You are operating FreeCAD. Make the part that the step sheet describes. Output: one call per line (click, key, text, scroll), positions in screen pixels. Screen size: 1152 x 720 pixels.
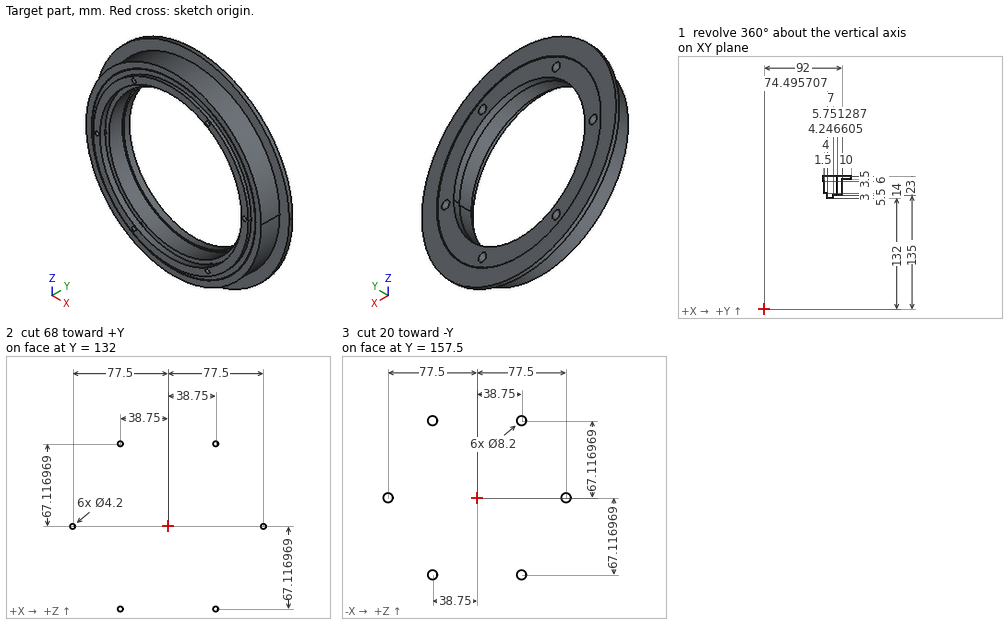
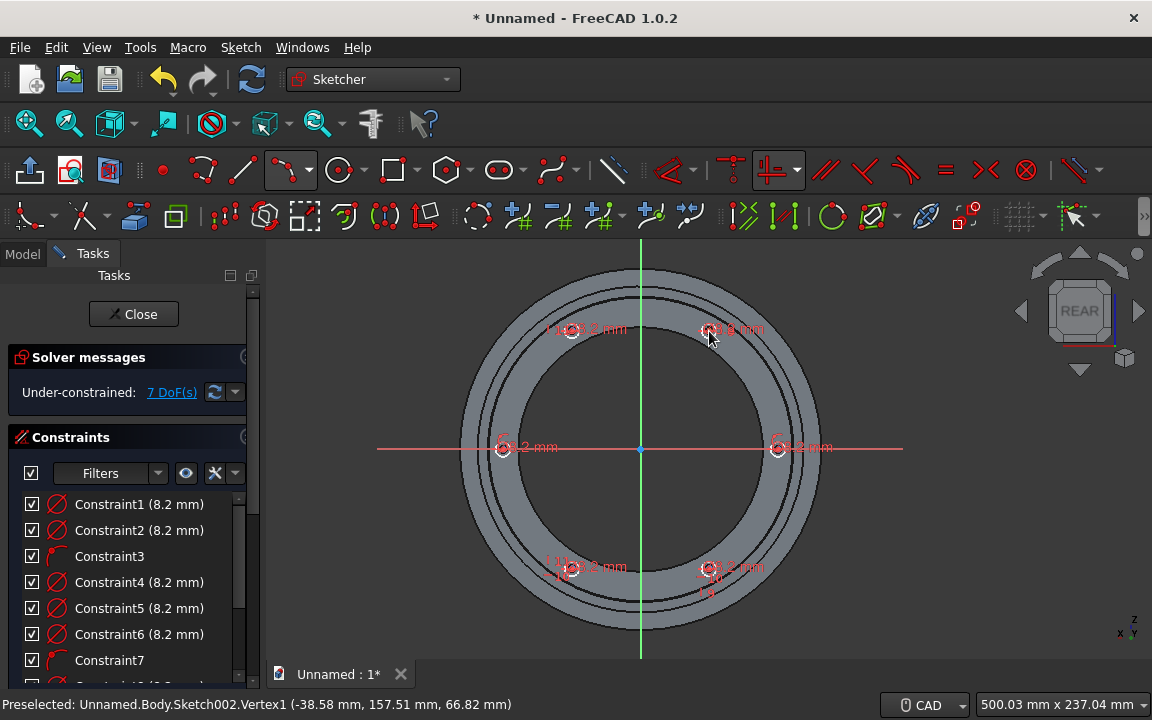
click(572, 331)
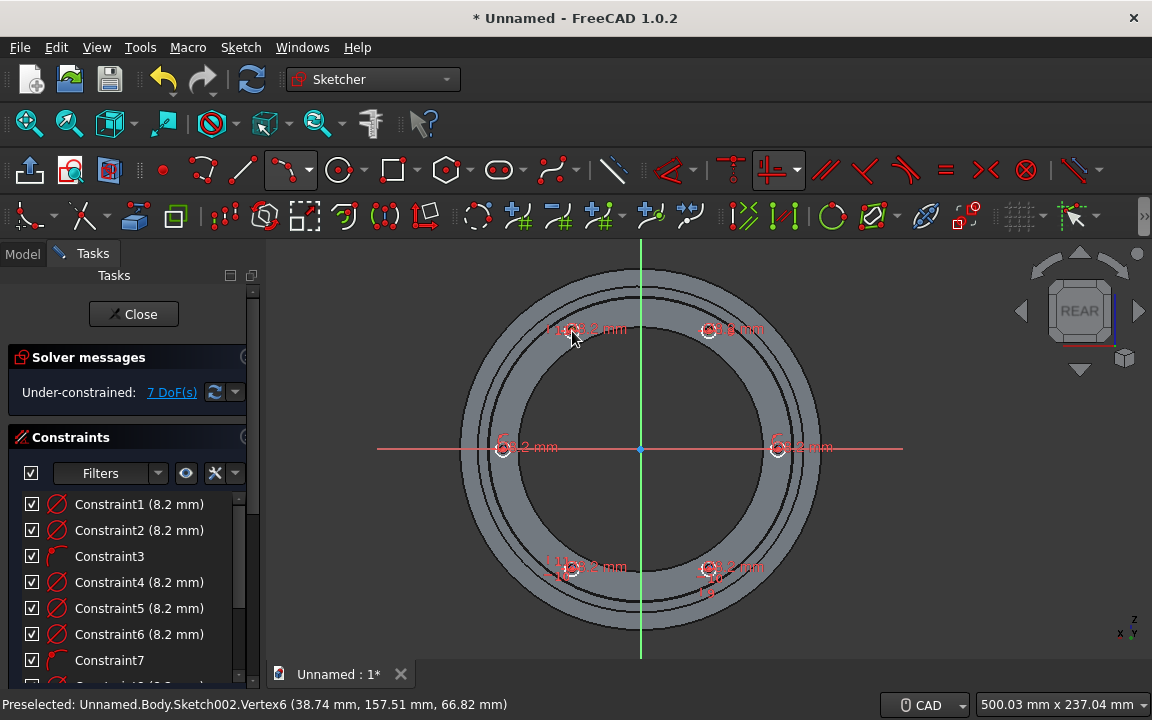
key(h)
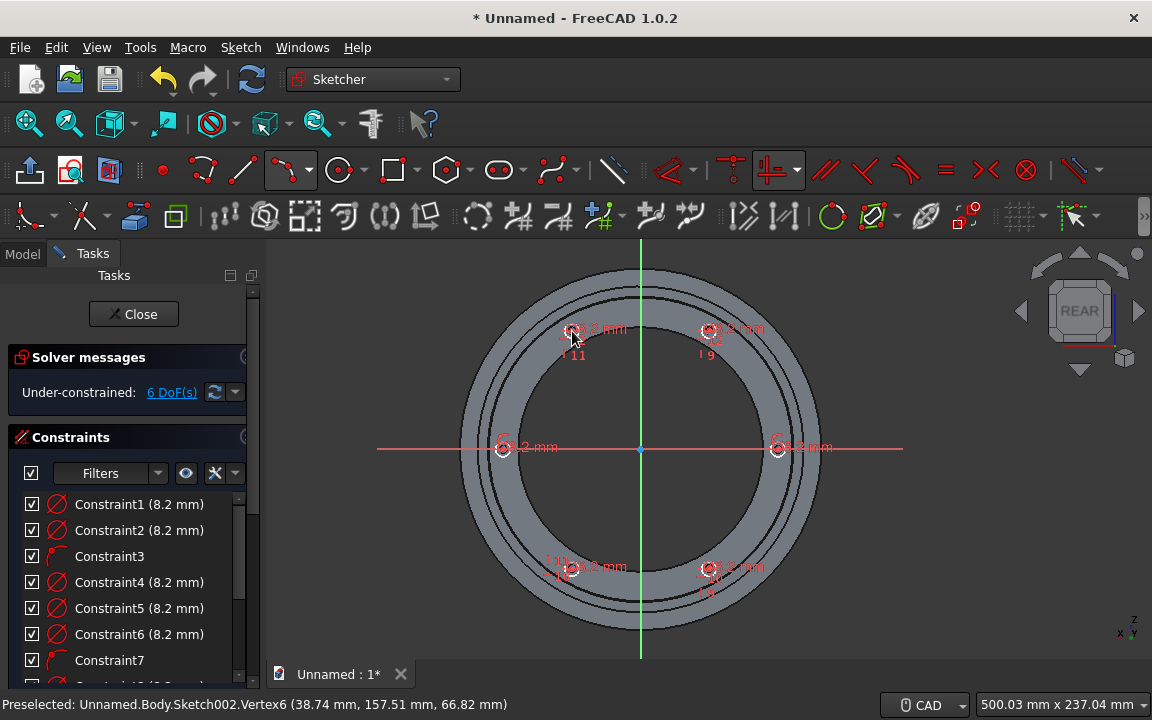
click(668, 170)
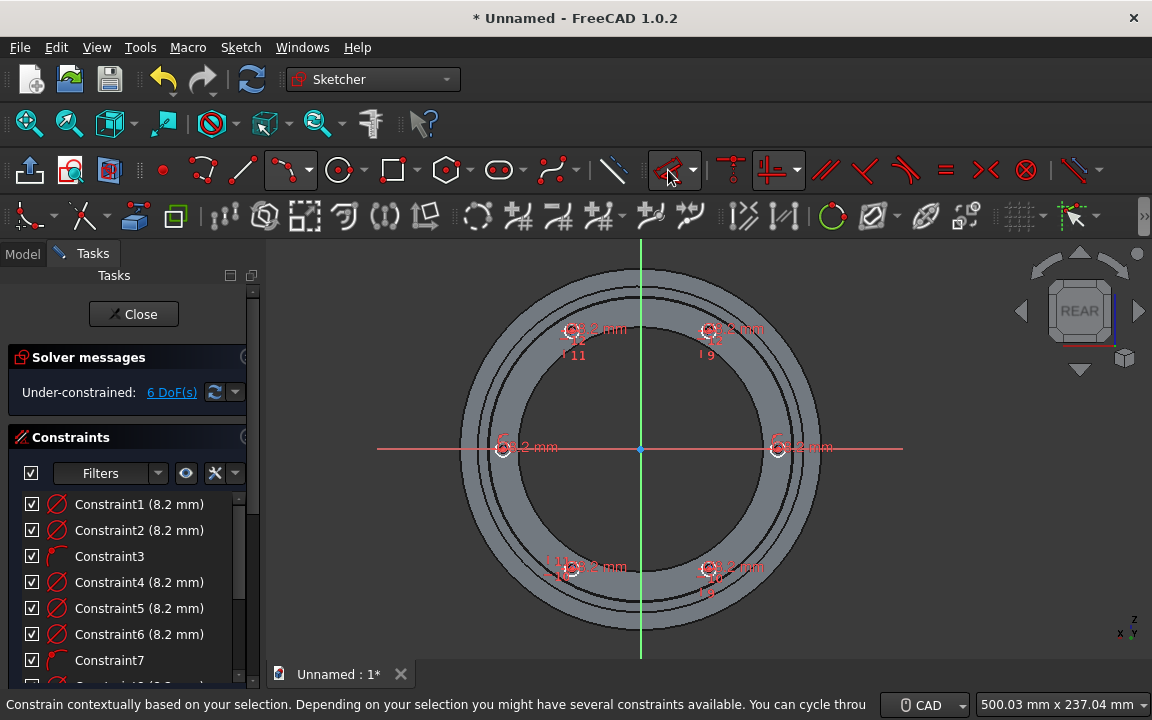
click(778, 449)
click(709, 483)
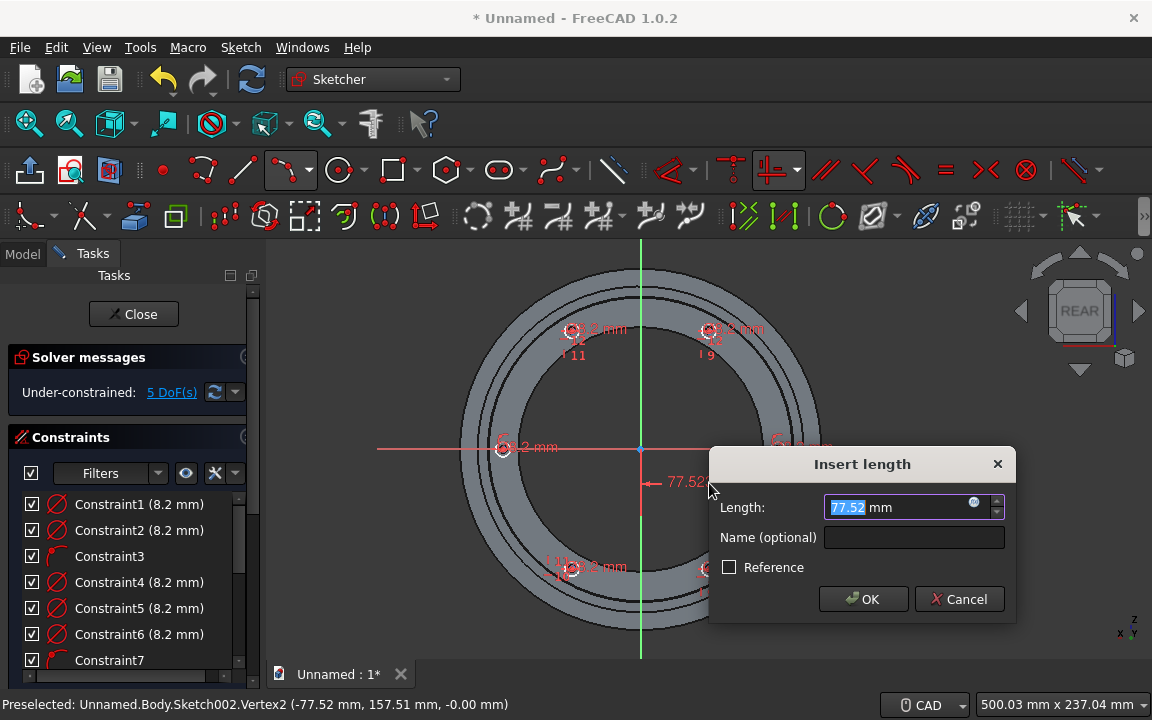
text(77.5)
key(Return)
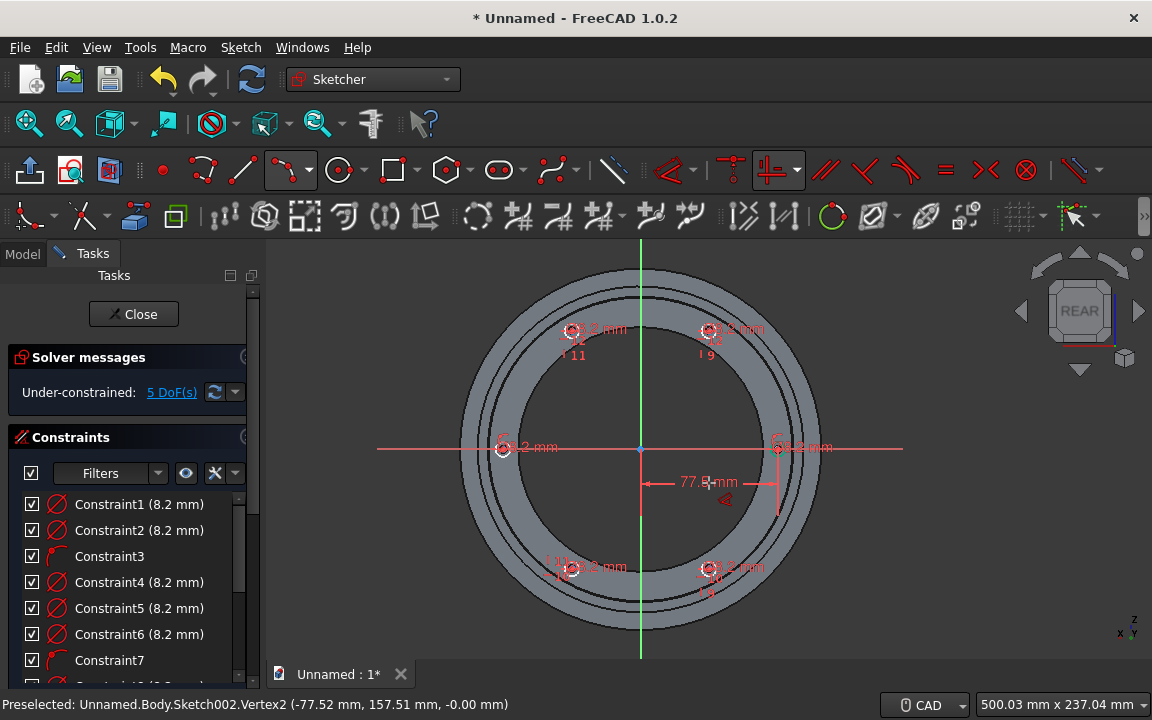
click(503, 449)
click(572, 483)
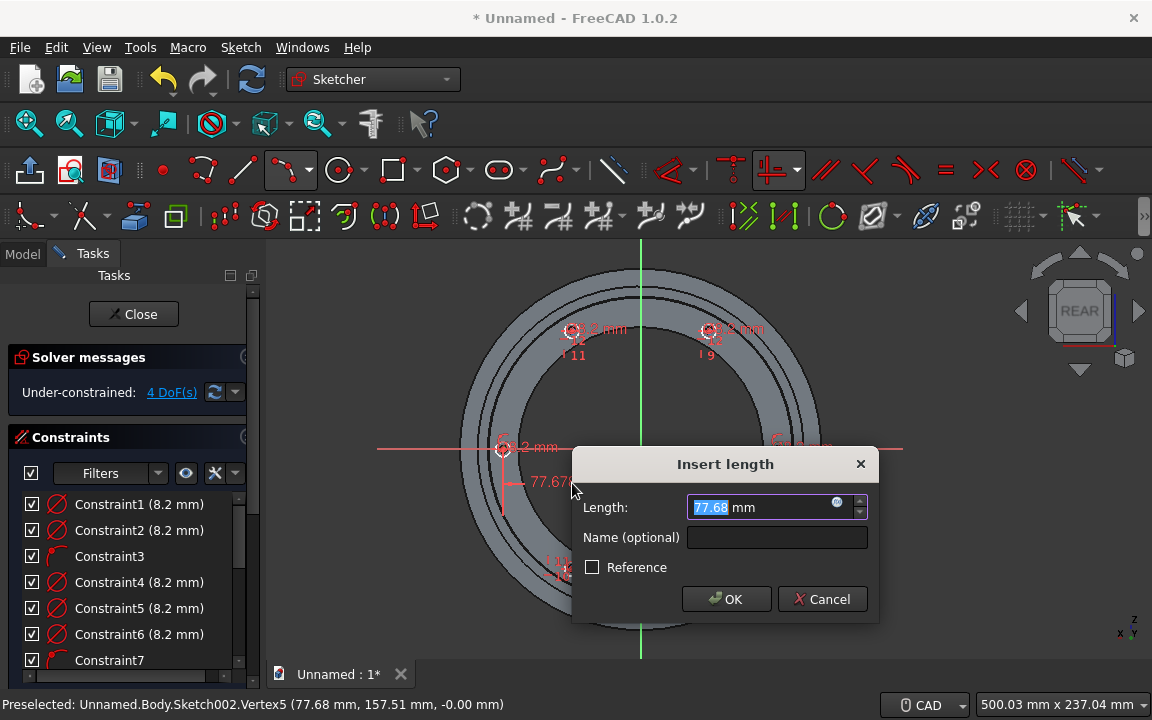
text(77.5)
key(Return)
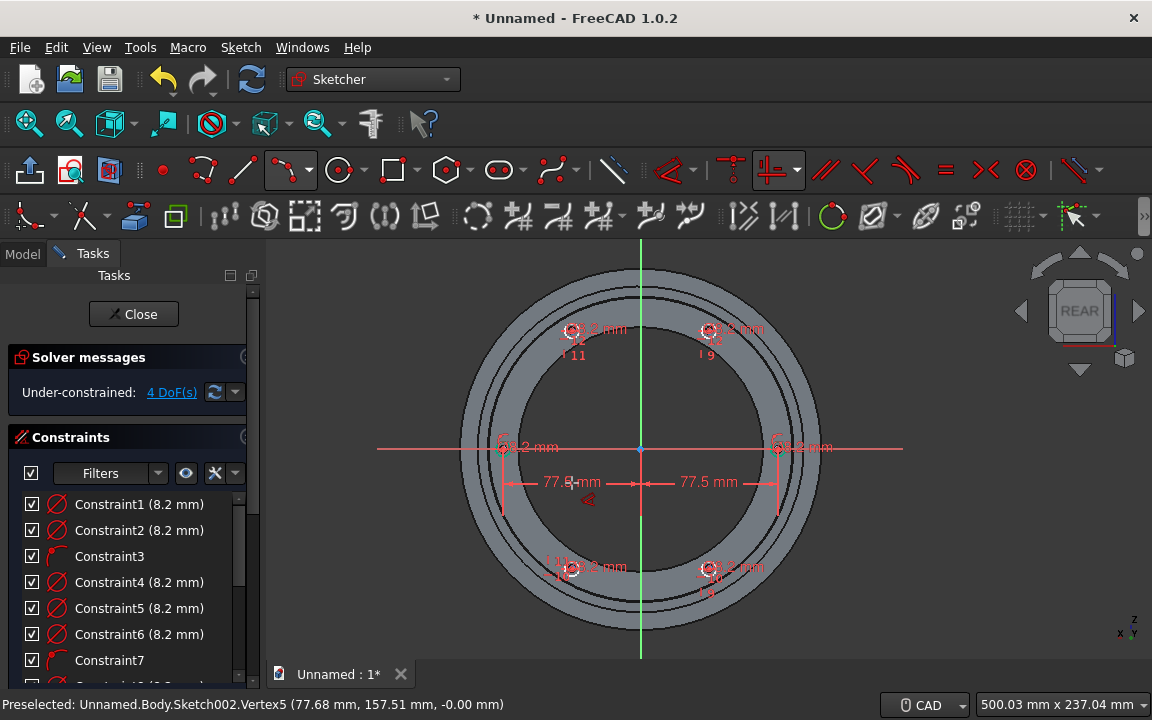
click(709, 331)
click(675, 297)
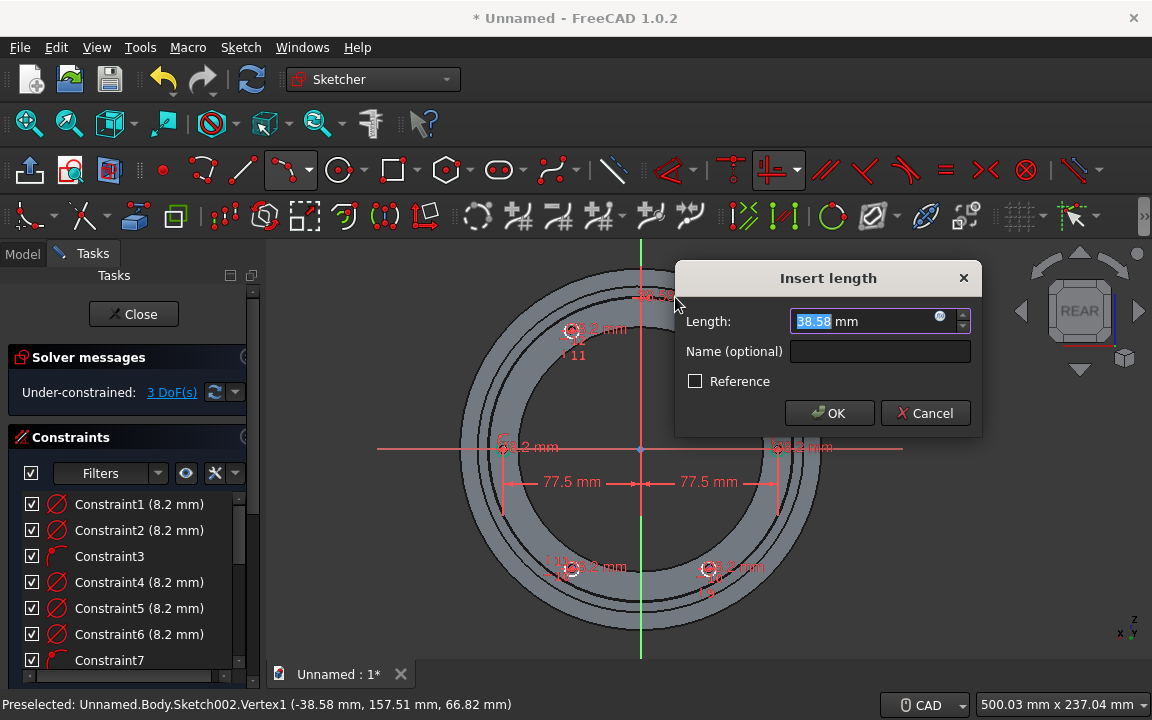
text(38.75)
key(Return)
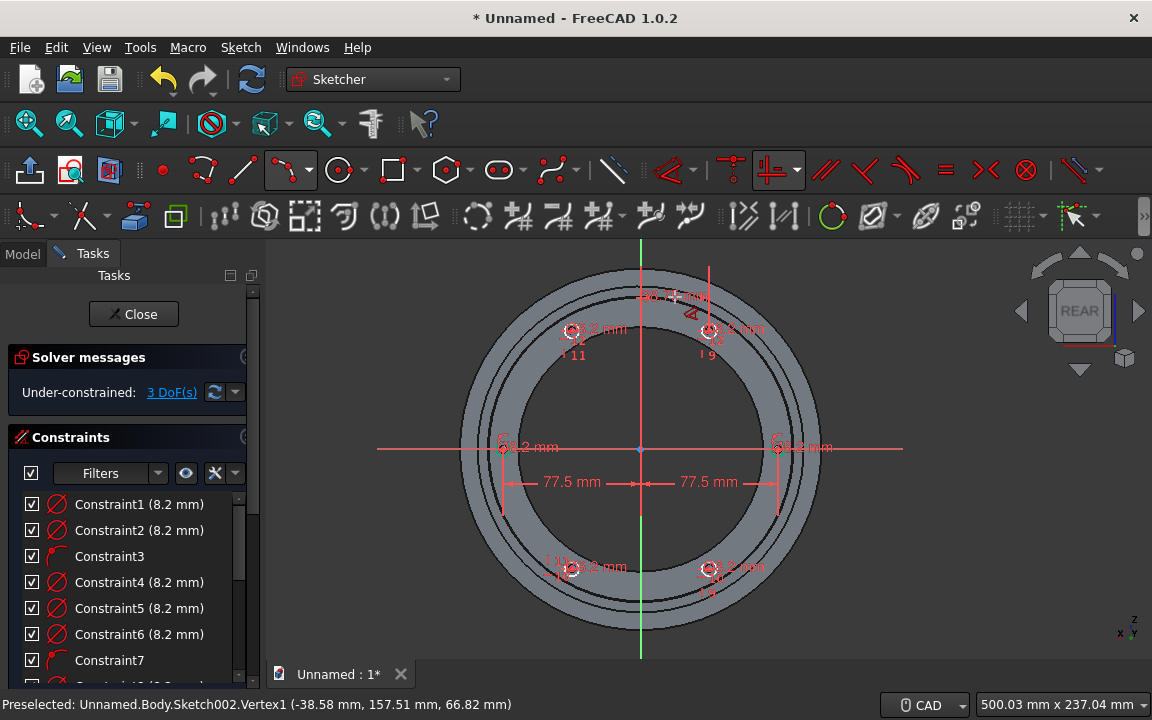
click(572, 569)
click(606, 603)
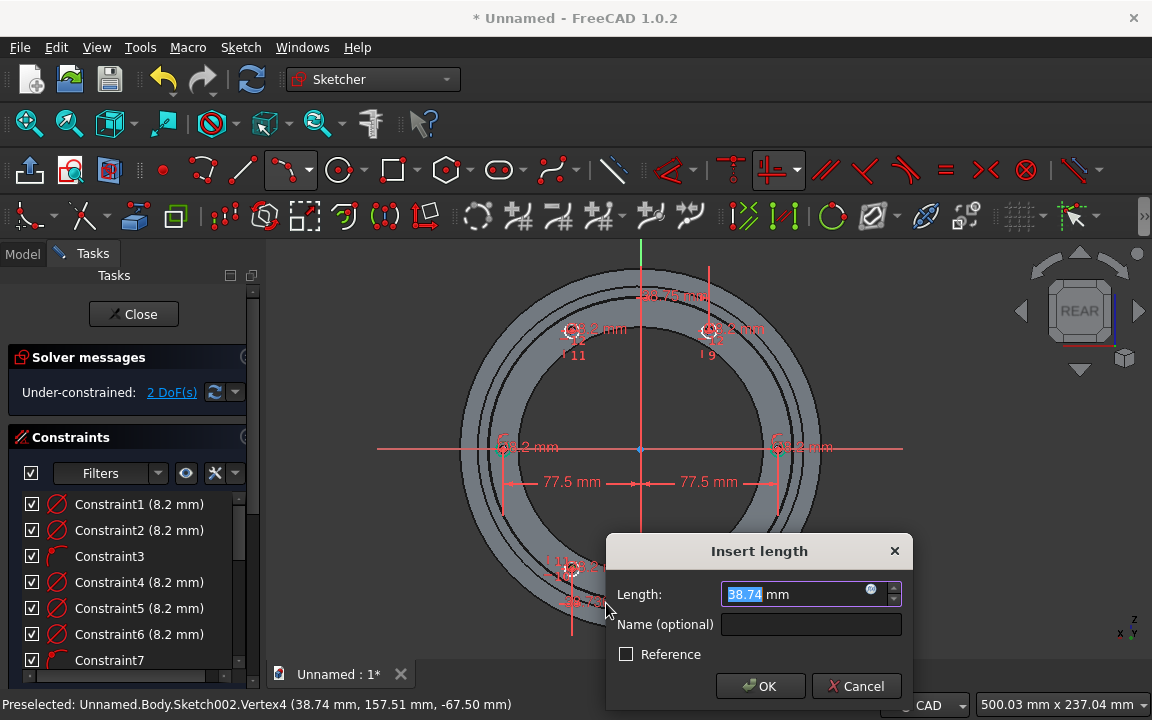
text(38.75)
key(Return)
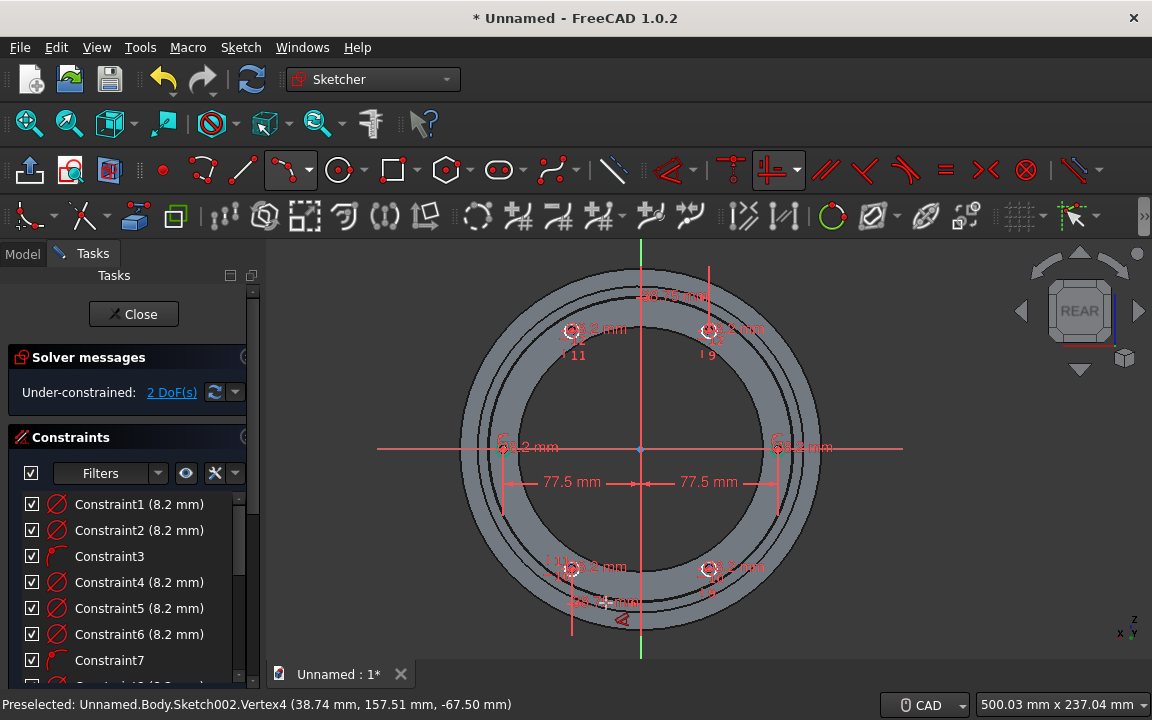
click(709, 331)
click(743, 390)